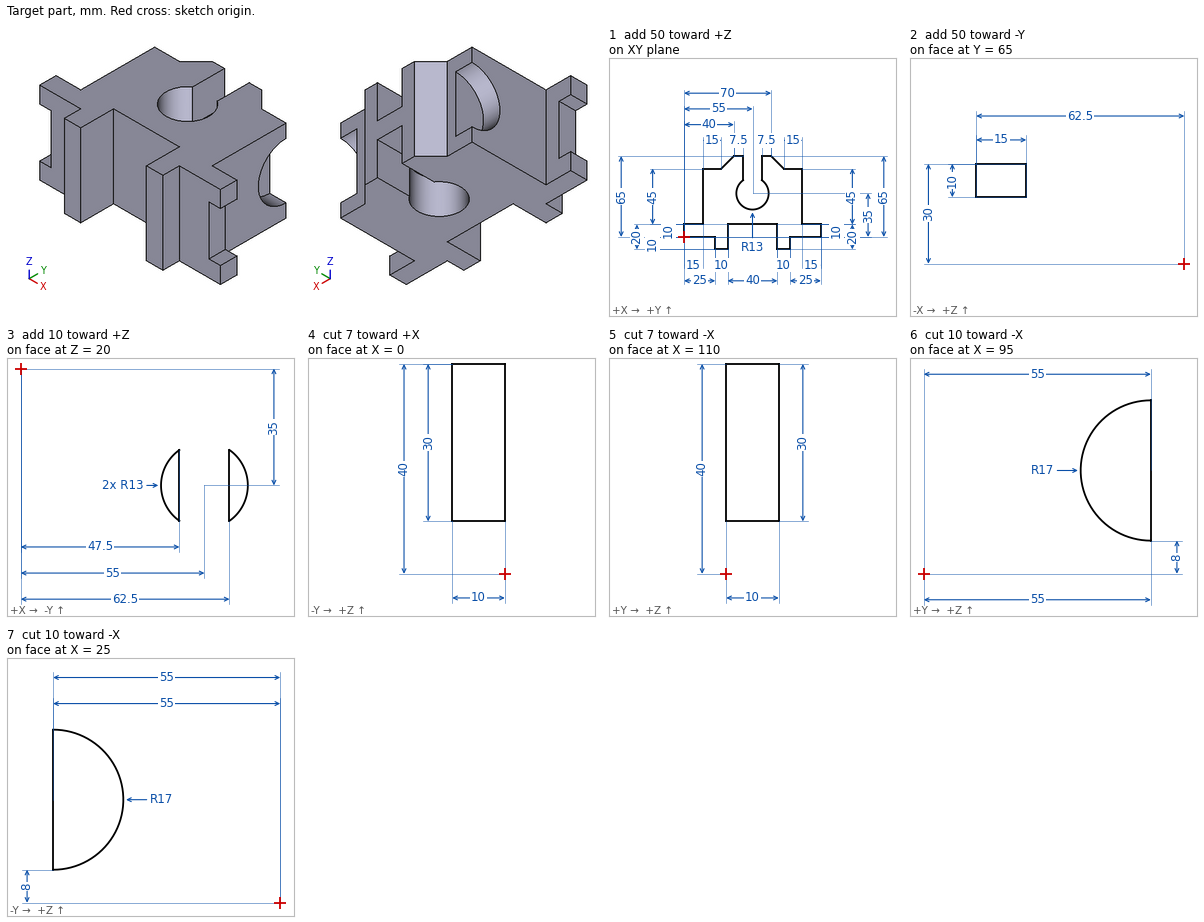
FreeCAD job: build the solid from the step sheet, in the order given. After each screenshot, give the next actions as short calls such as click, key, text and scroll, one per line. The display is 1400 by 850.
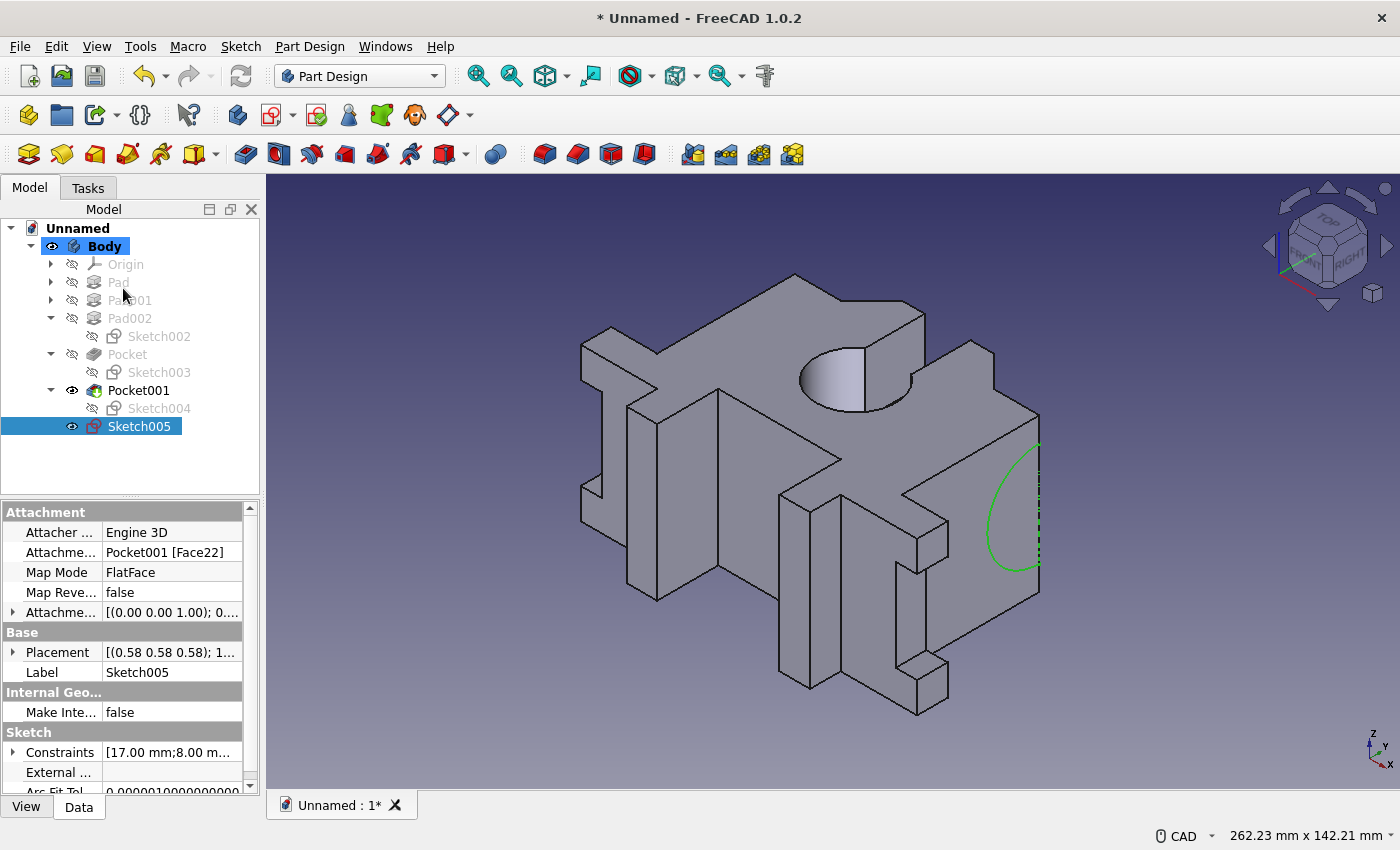
click(246, 154)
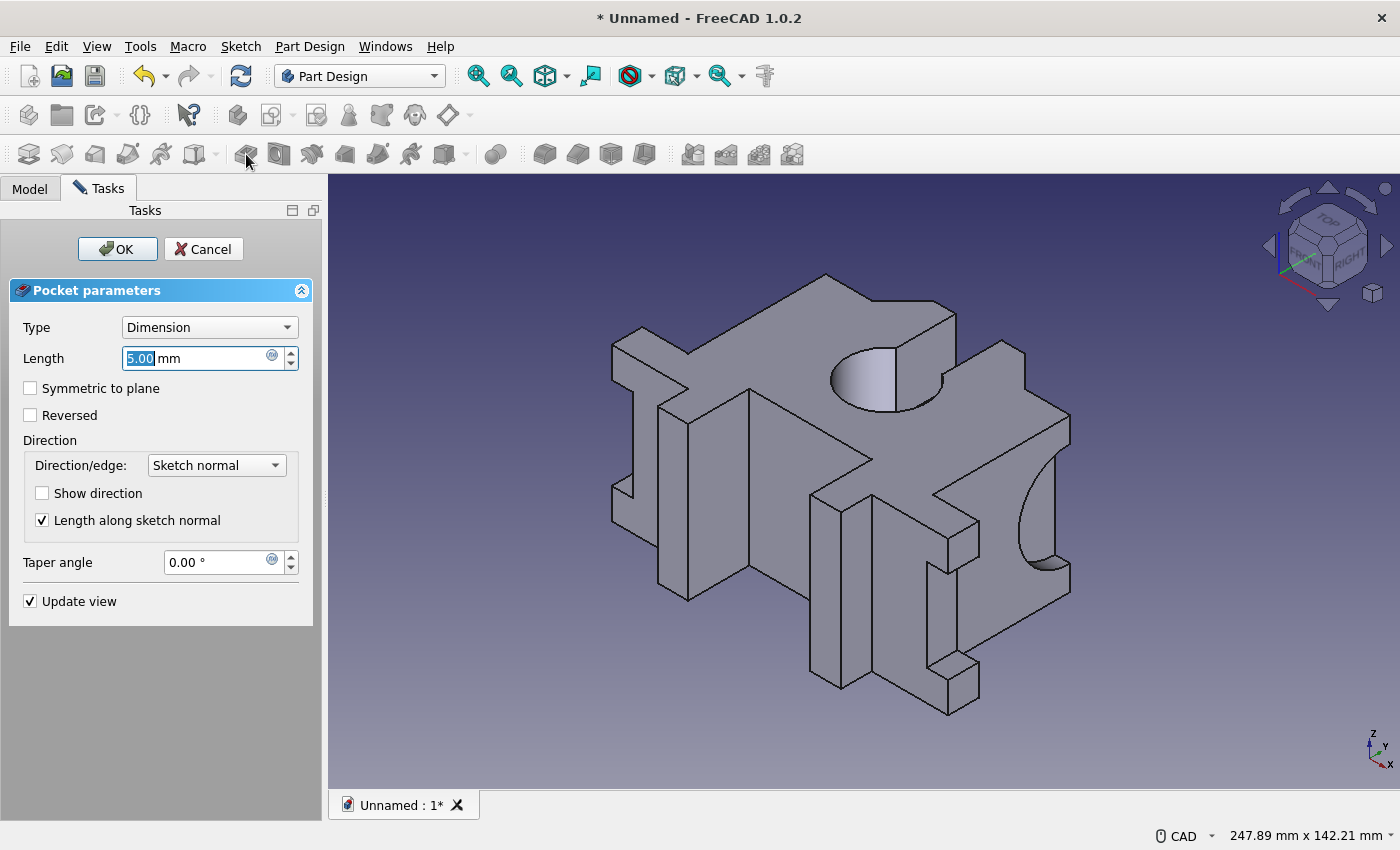
text(10)
key(Tab)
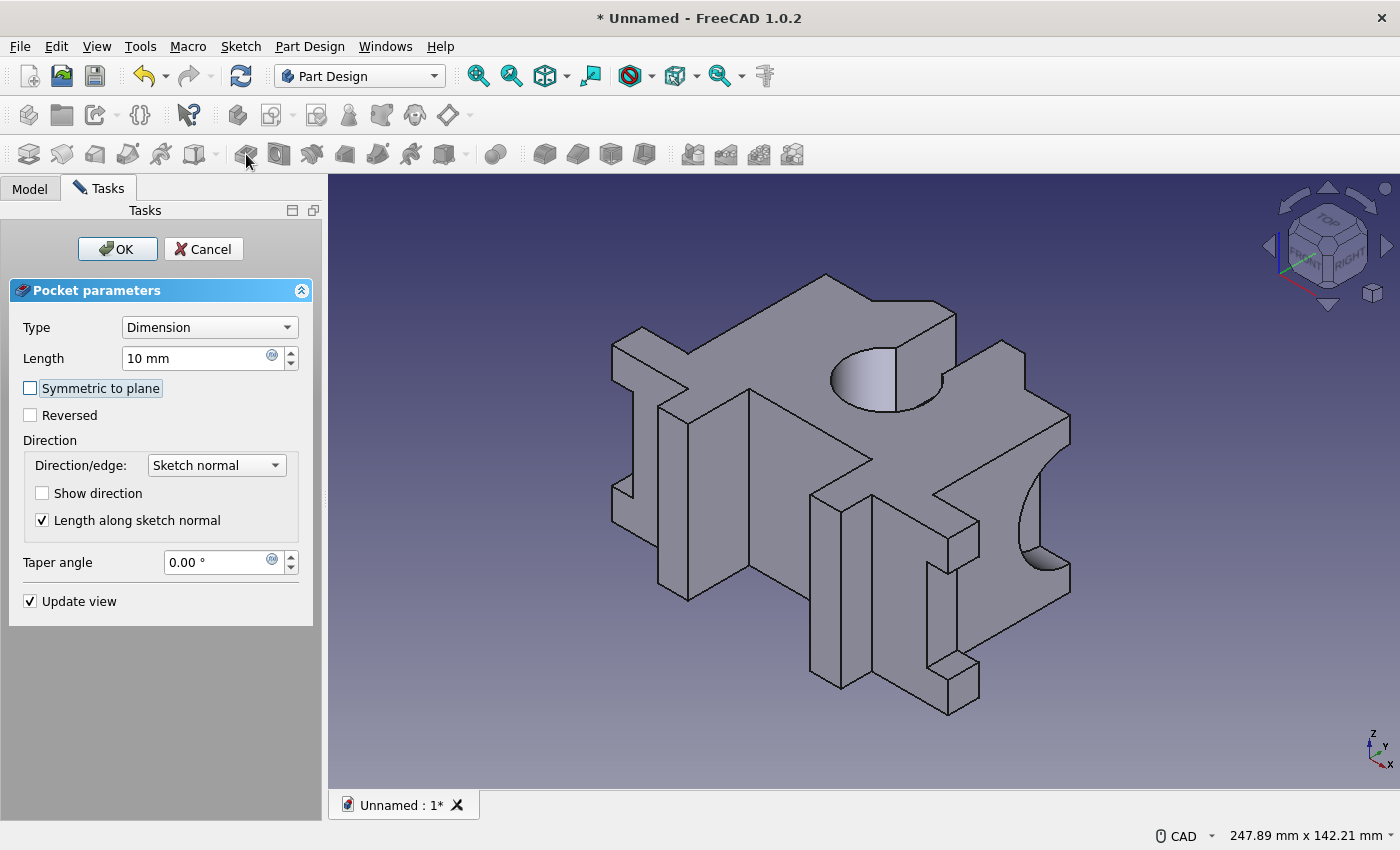
click(118, 249)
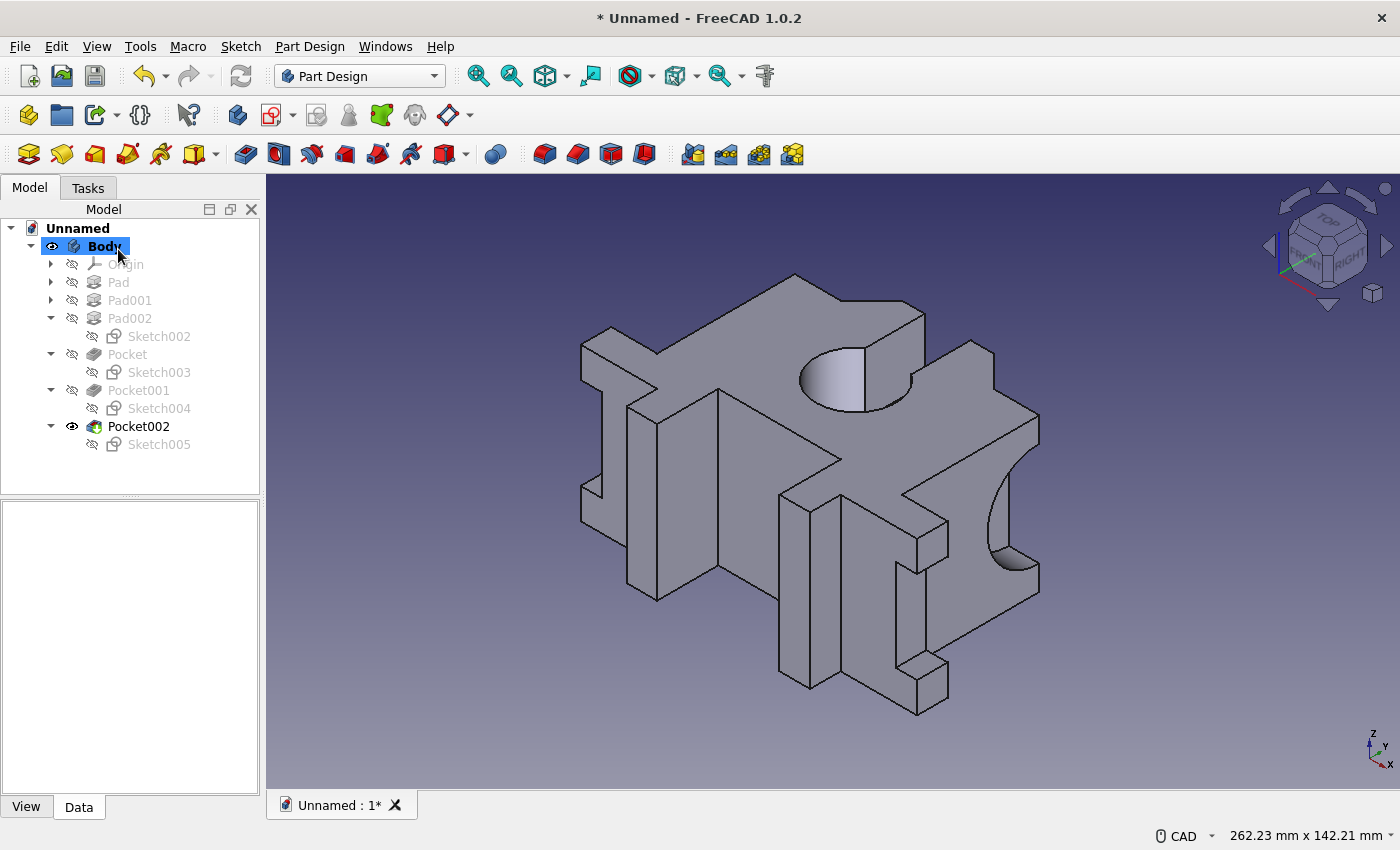
key(6)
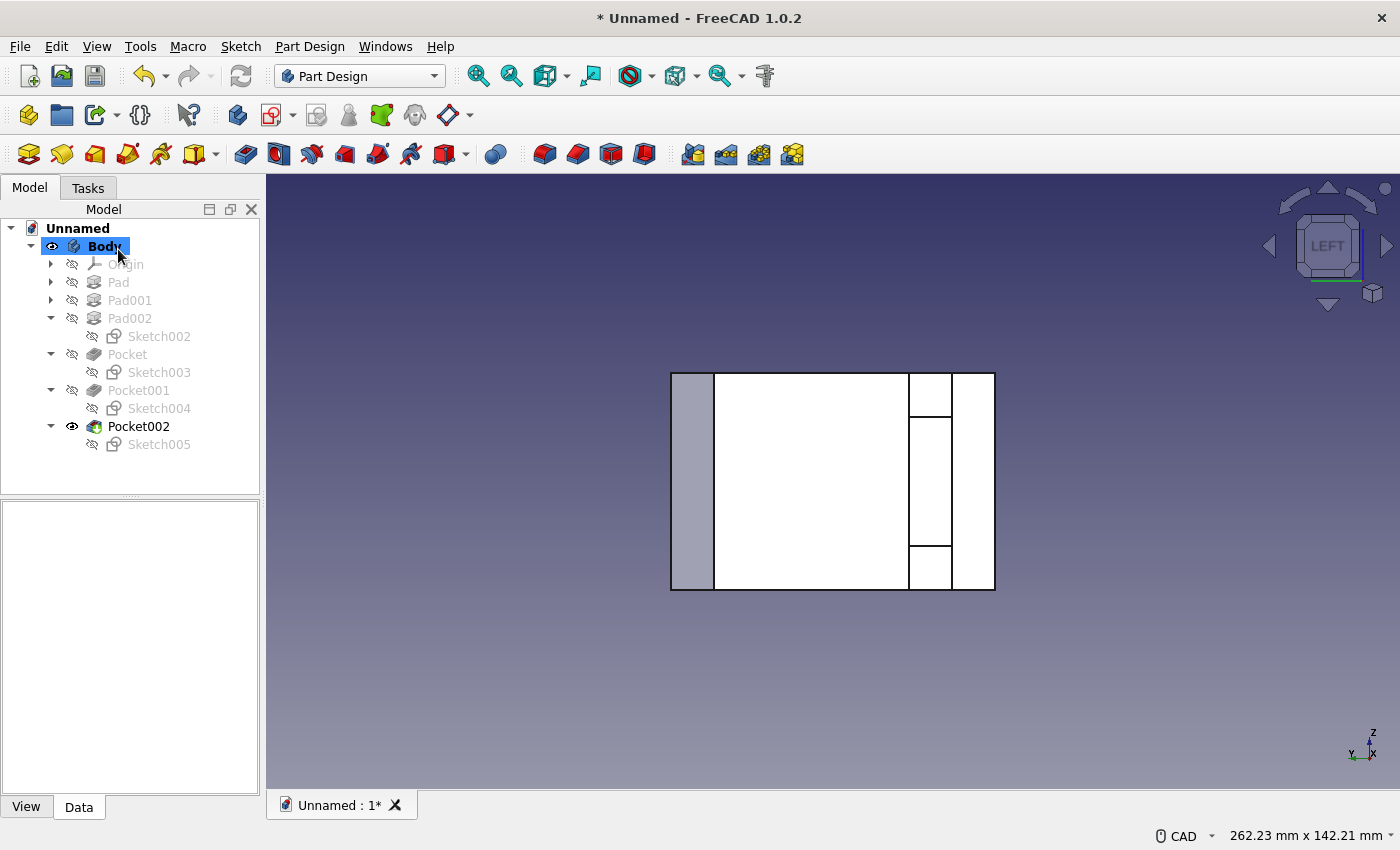
click(479, 76)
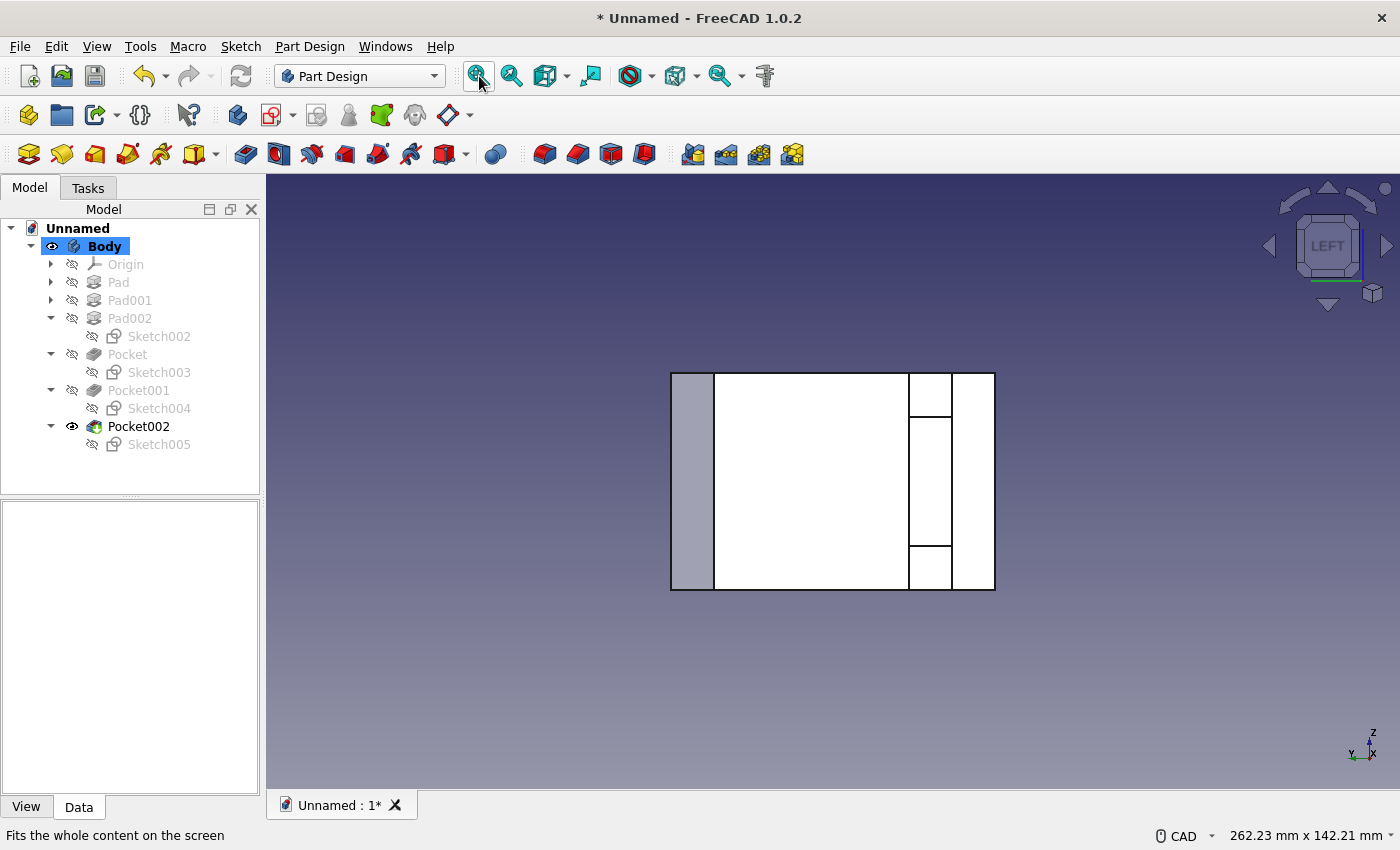
click(974, 419)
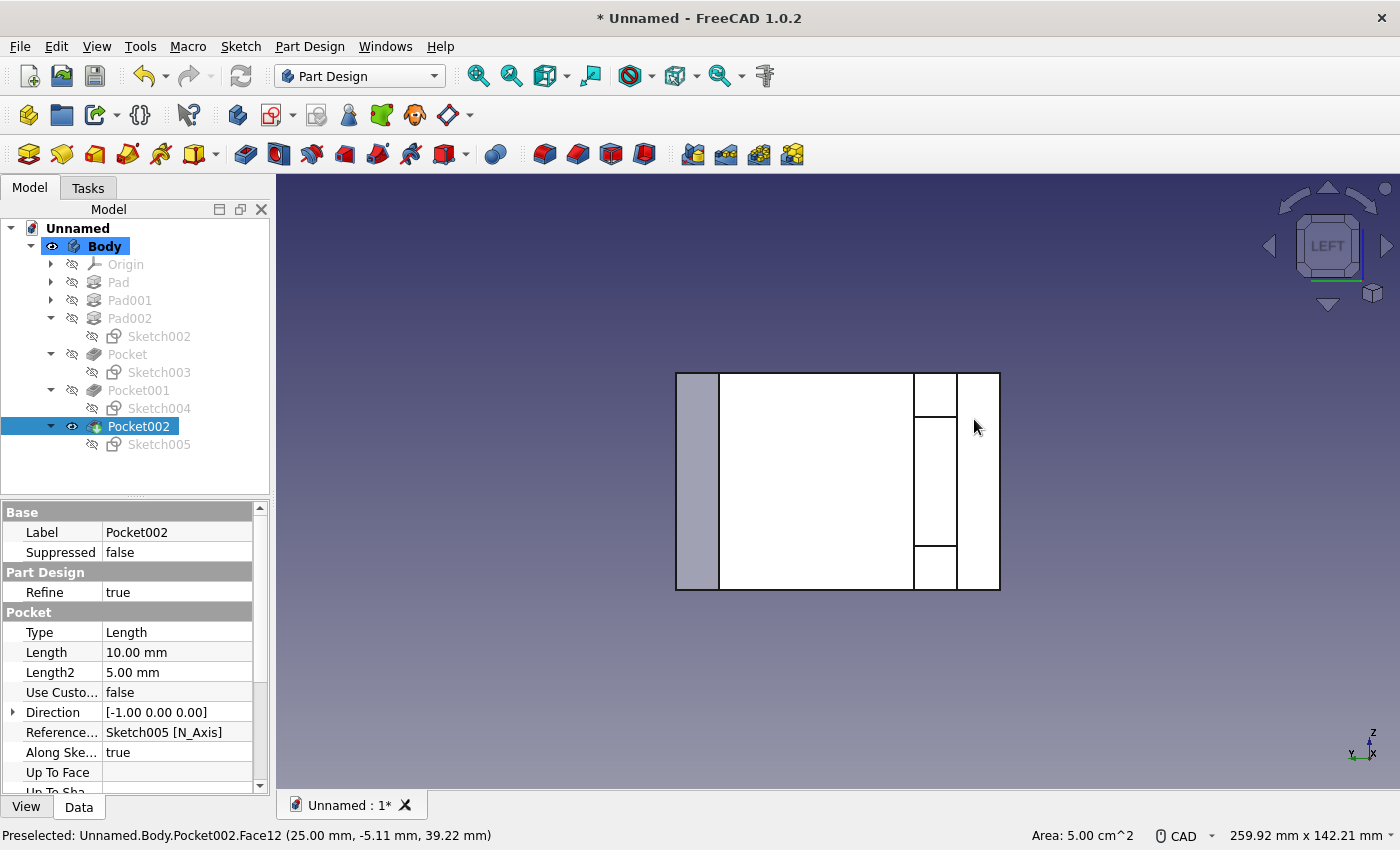
click(270, 116)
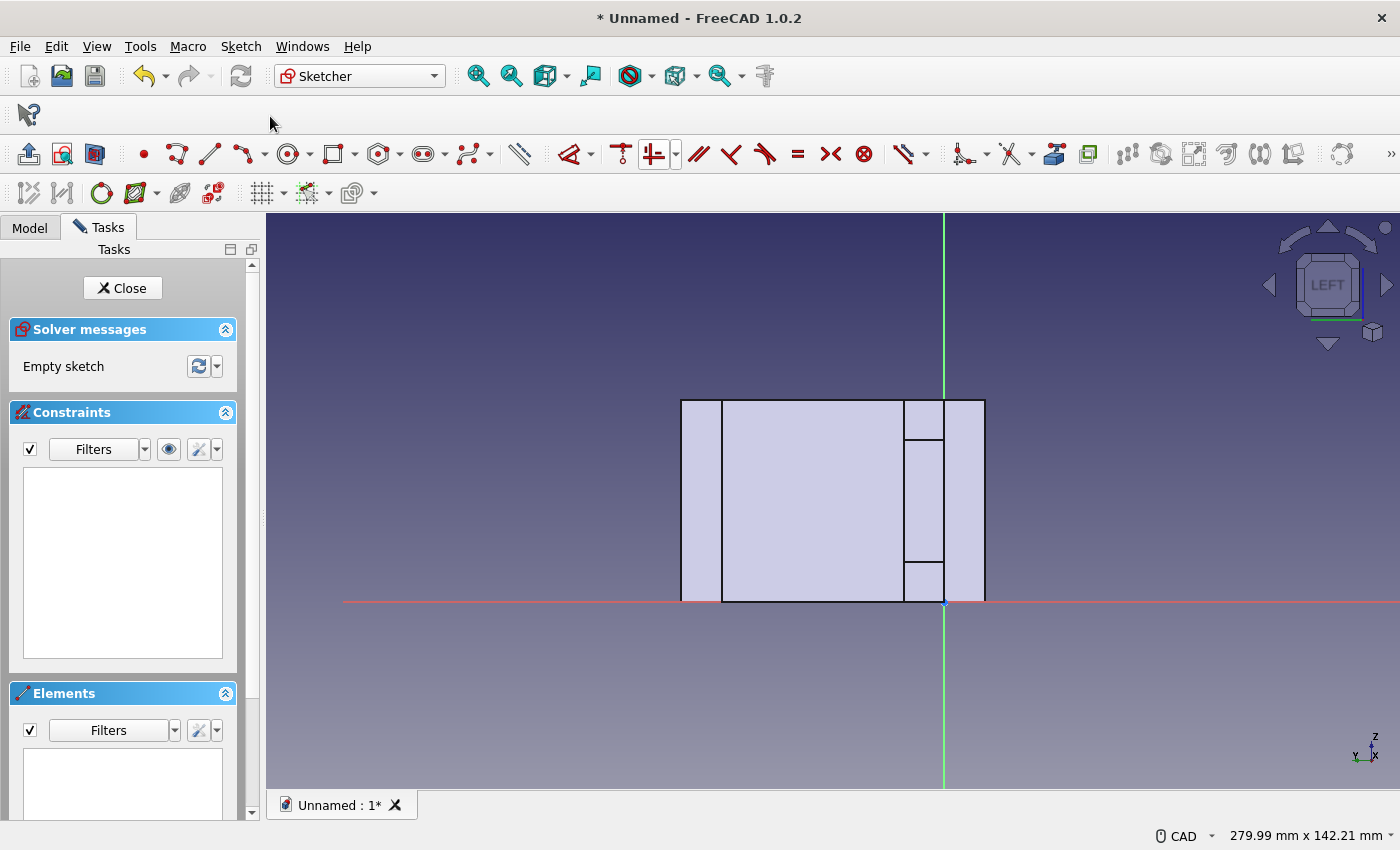
scroll(889, 530, up, 4)